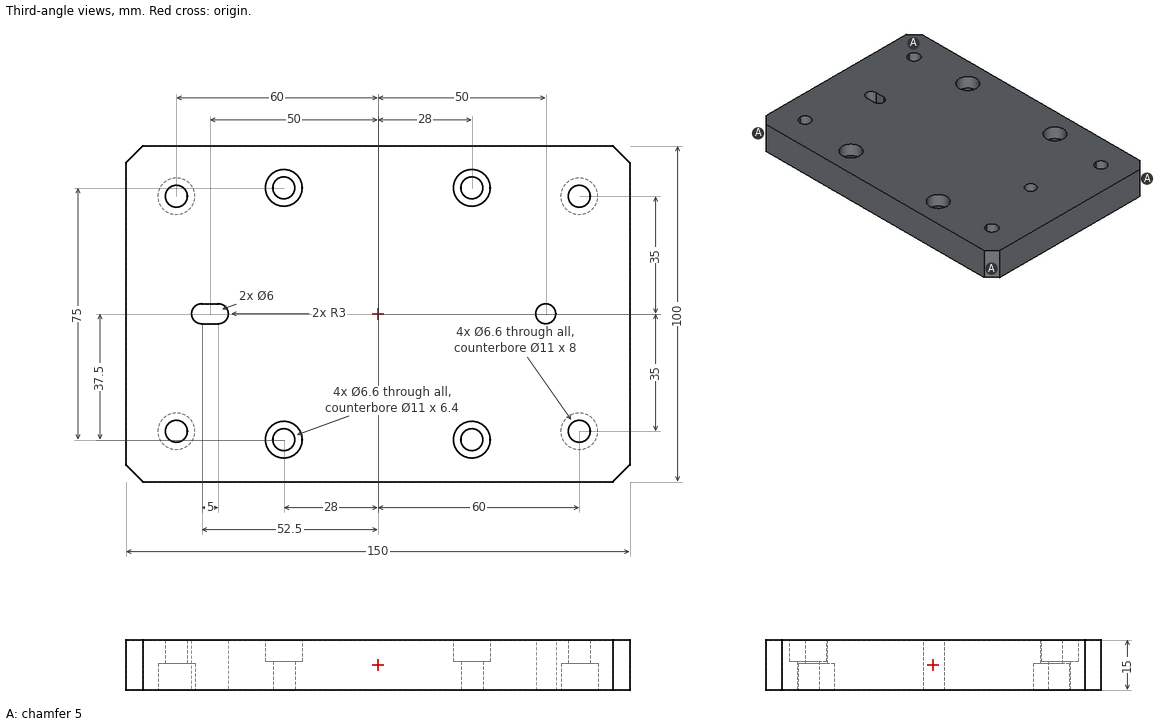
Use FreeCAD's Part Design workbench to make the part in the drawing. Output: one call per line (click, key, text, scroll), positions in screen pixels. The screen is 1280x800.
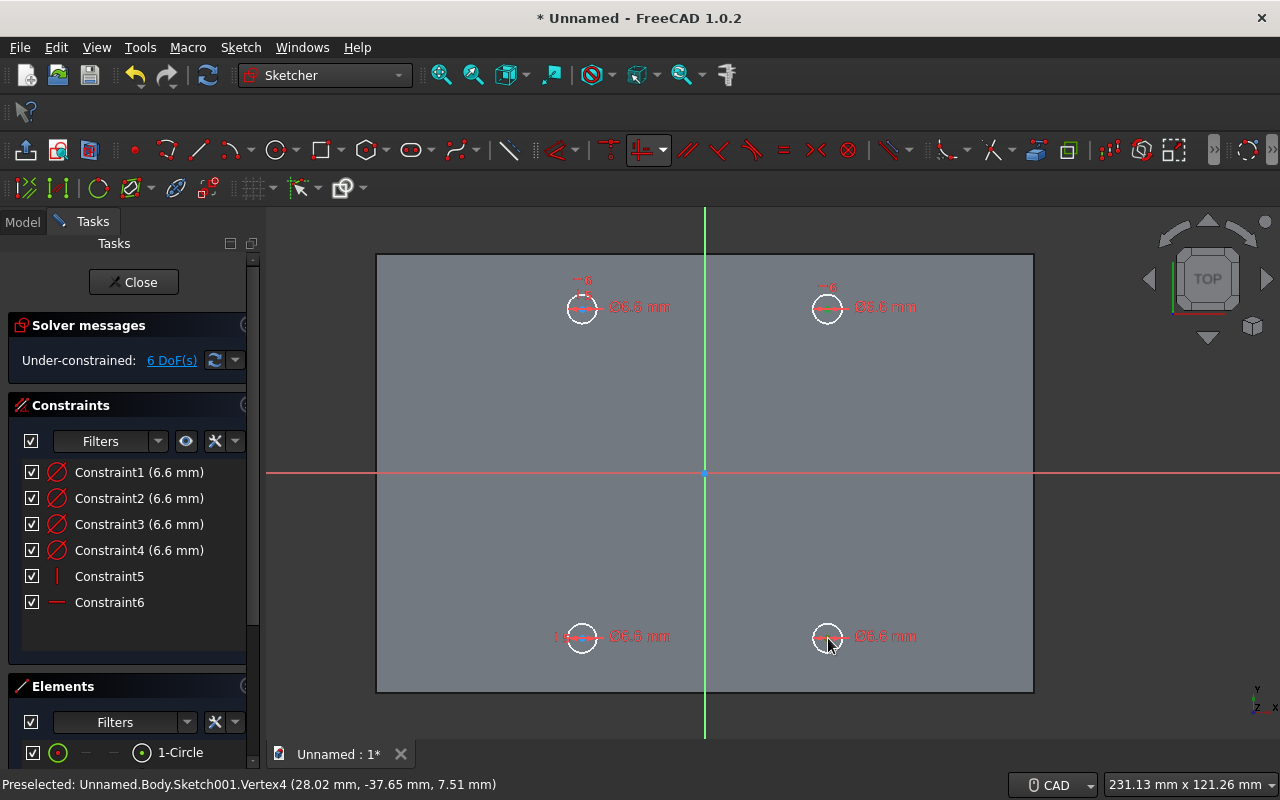
click(666, 150)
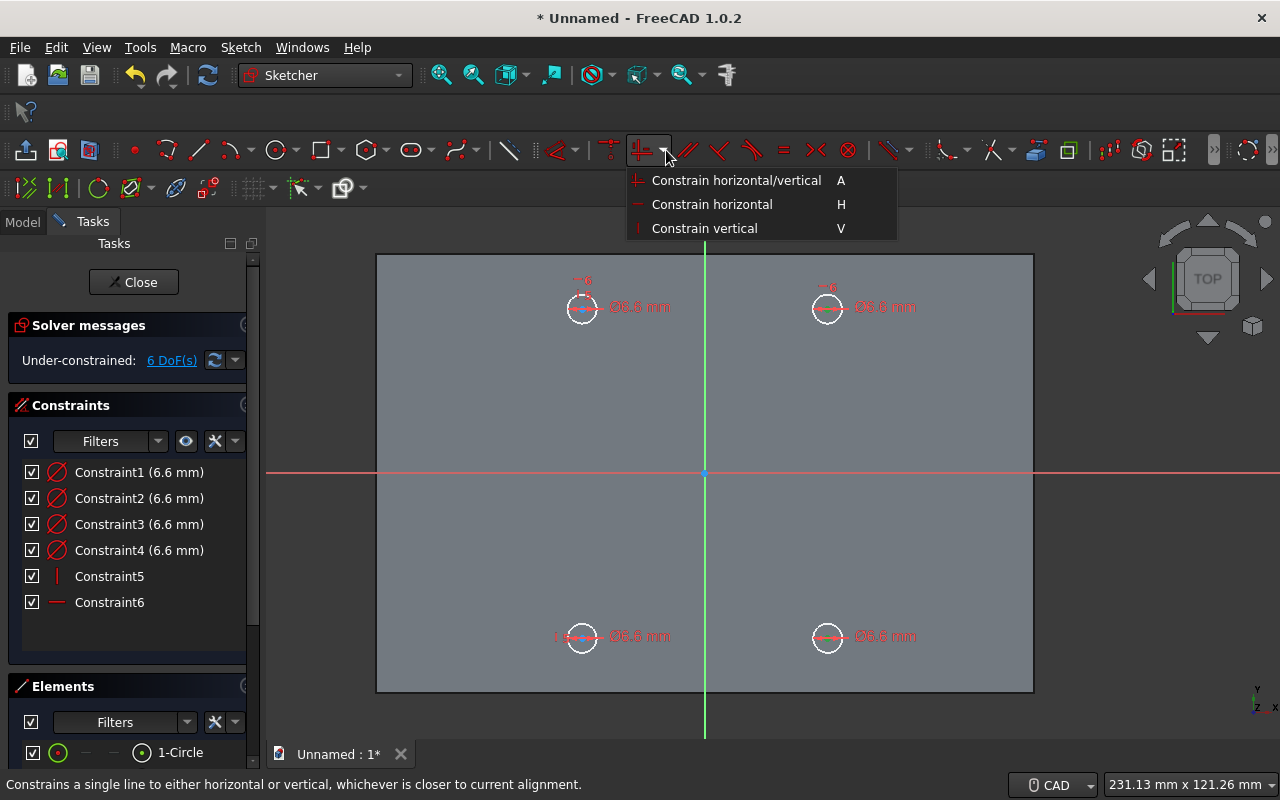
click(762, 228)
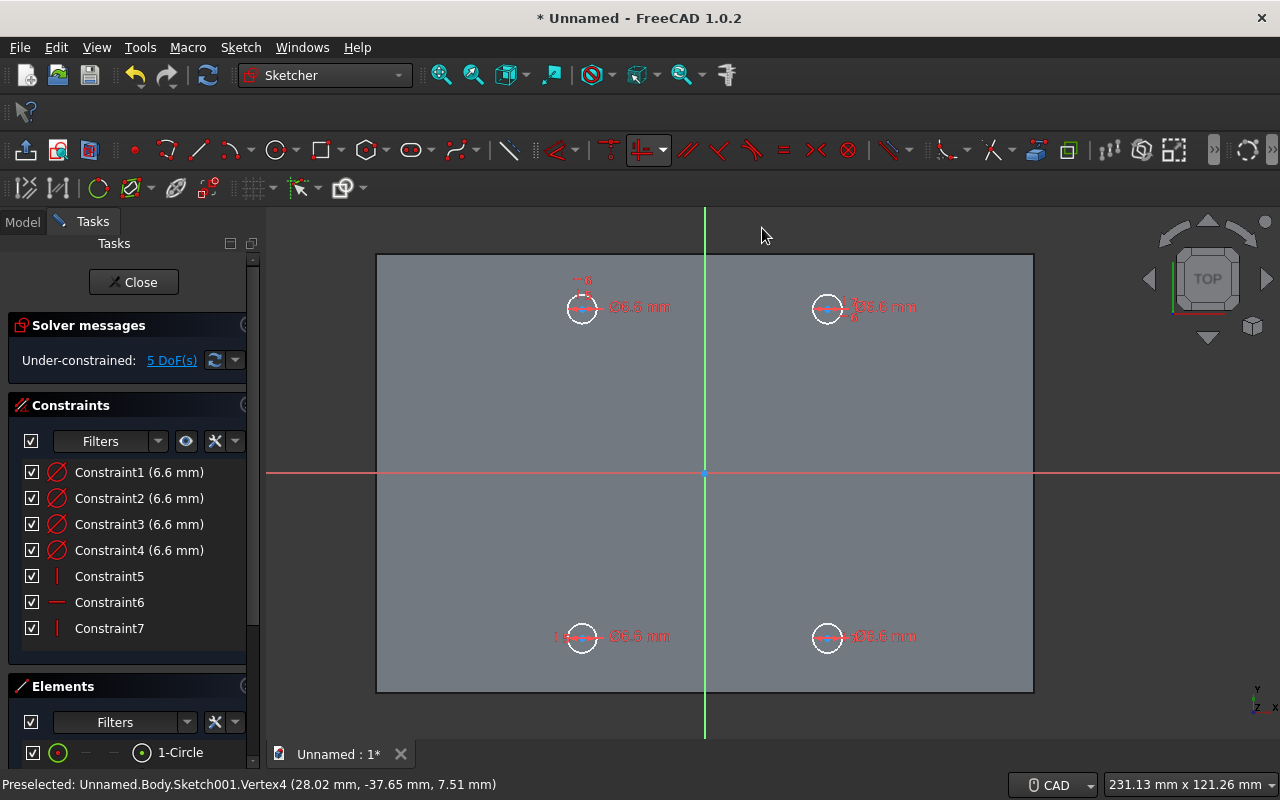
click(582, 638)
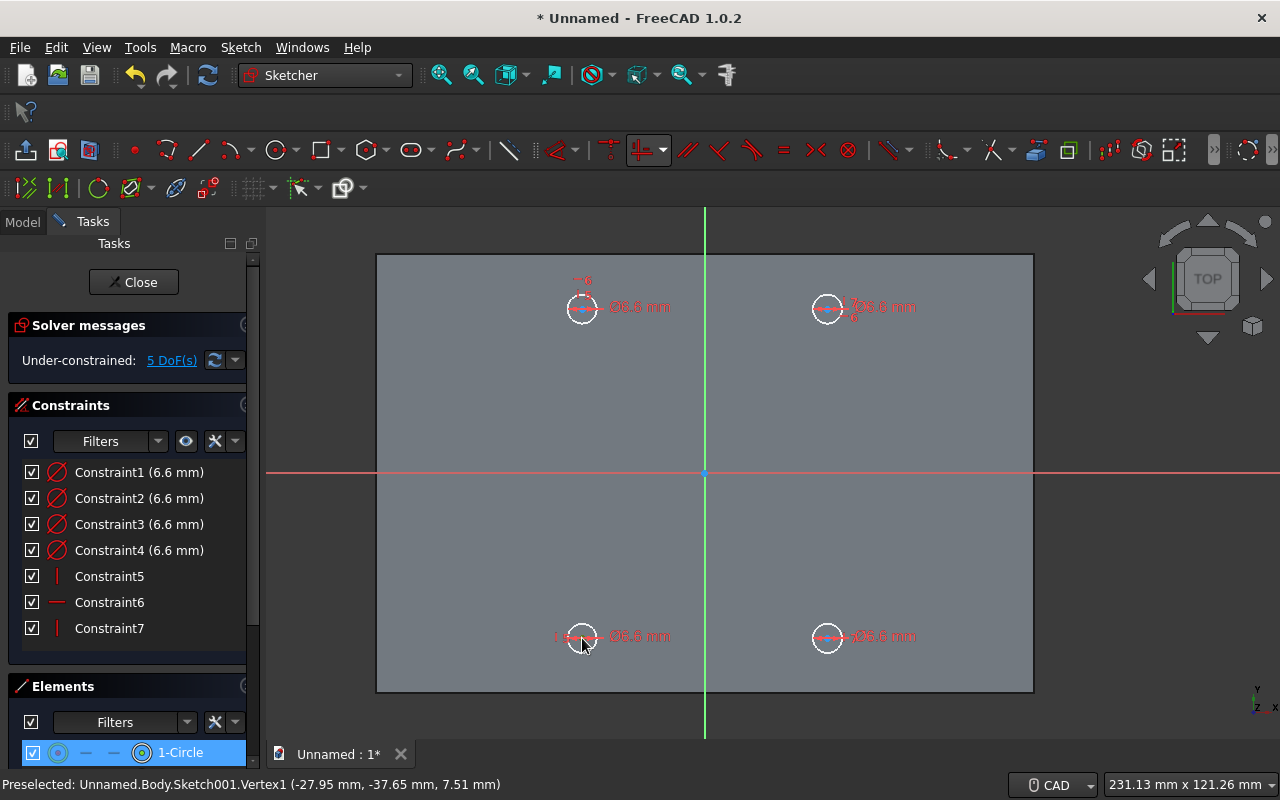
click(827, 638)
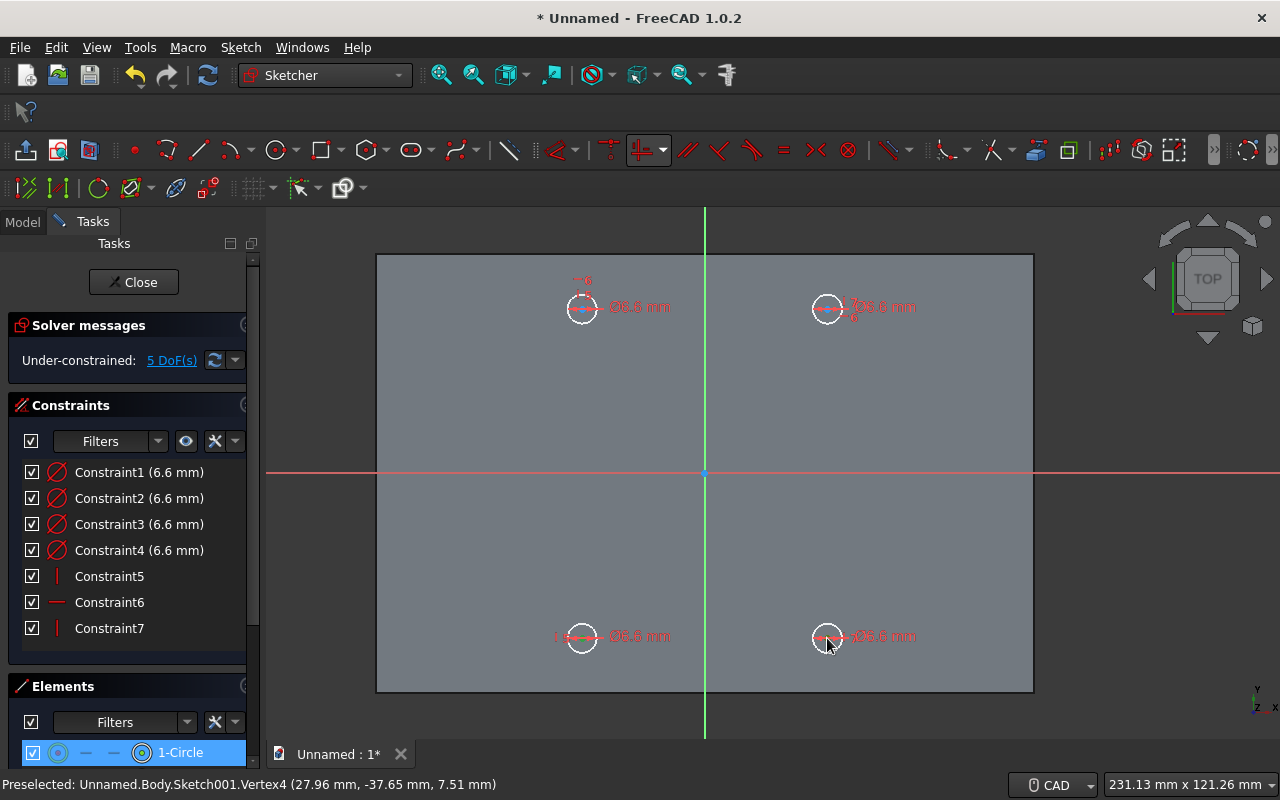
key(h)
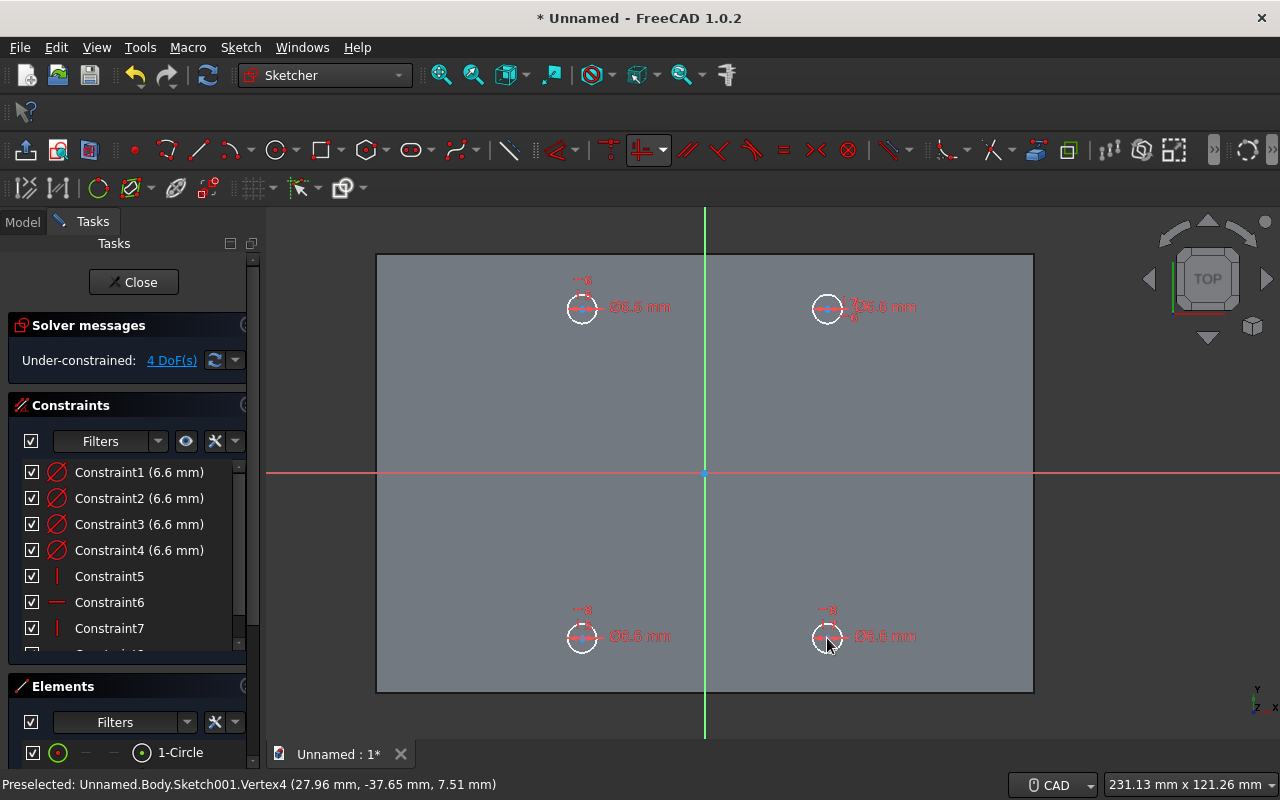
key(d)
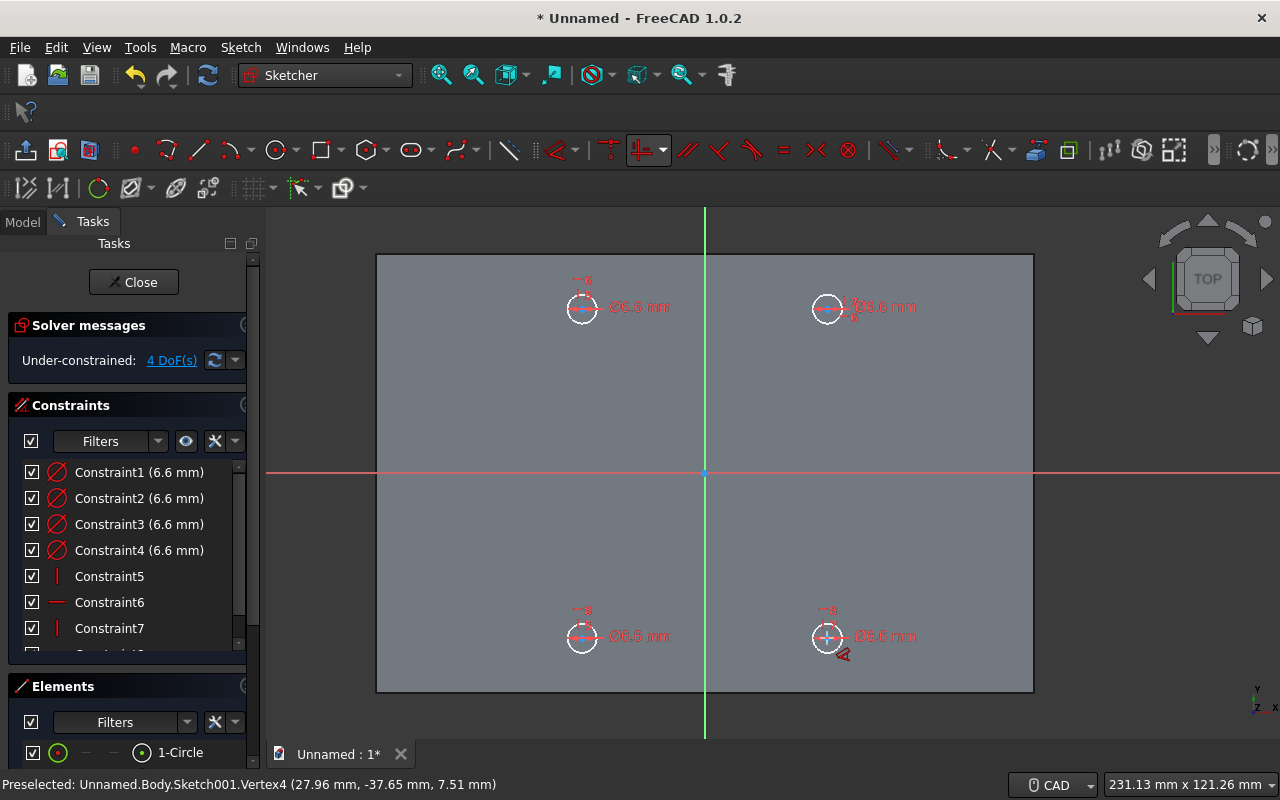
click(582, 638)
click(643, 672)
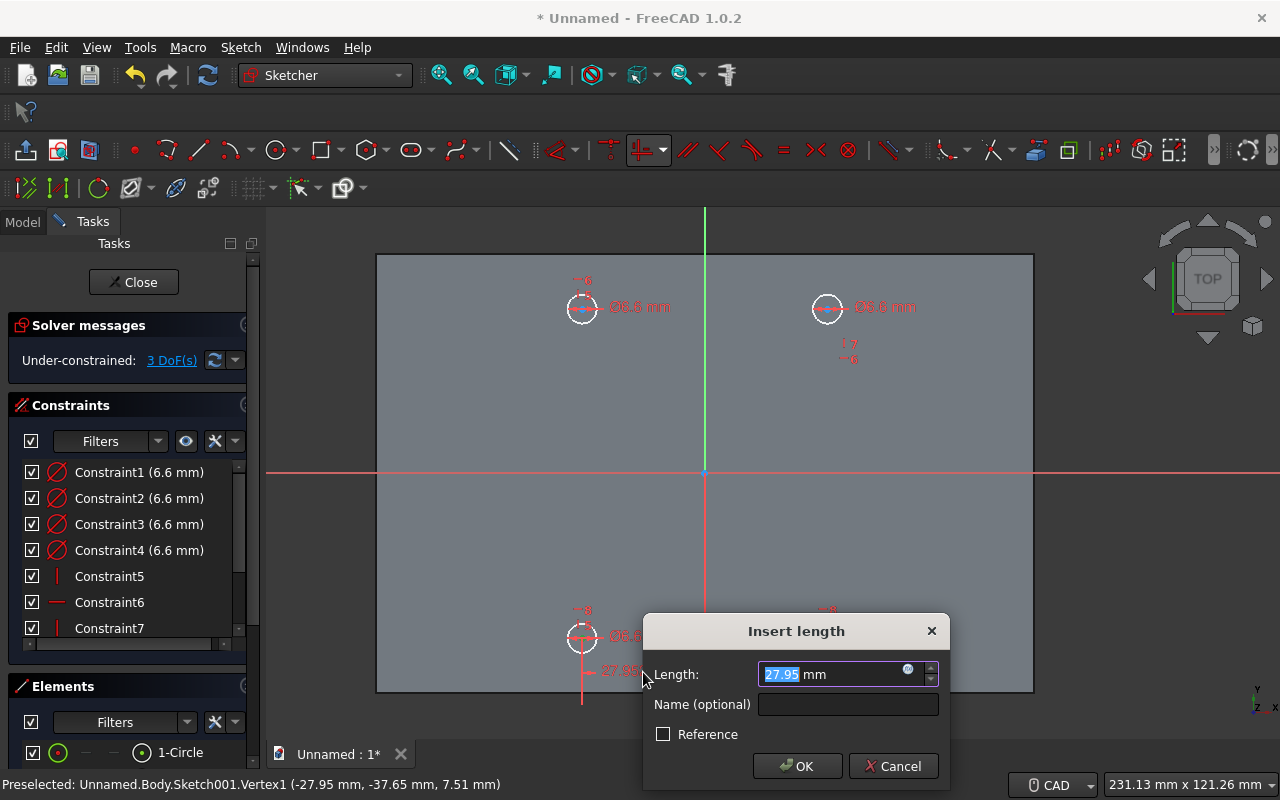
text(28)
key(Return)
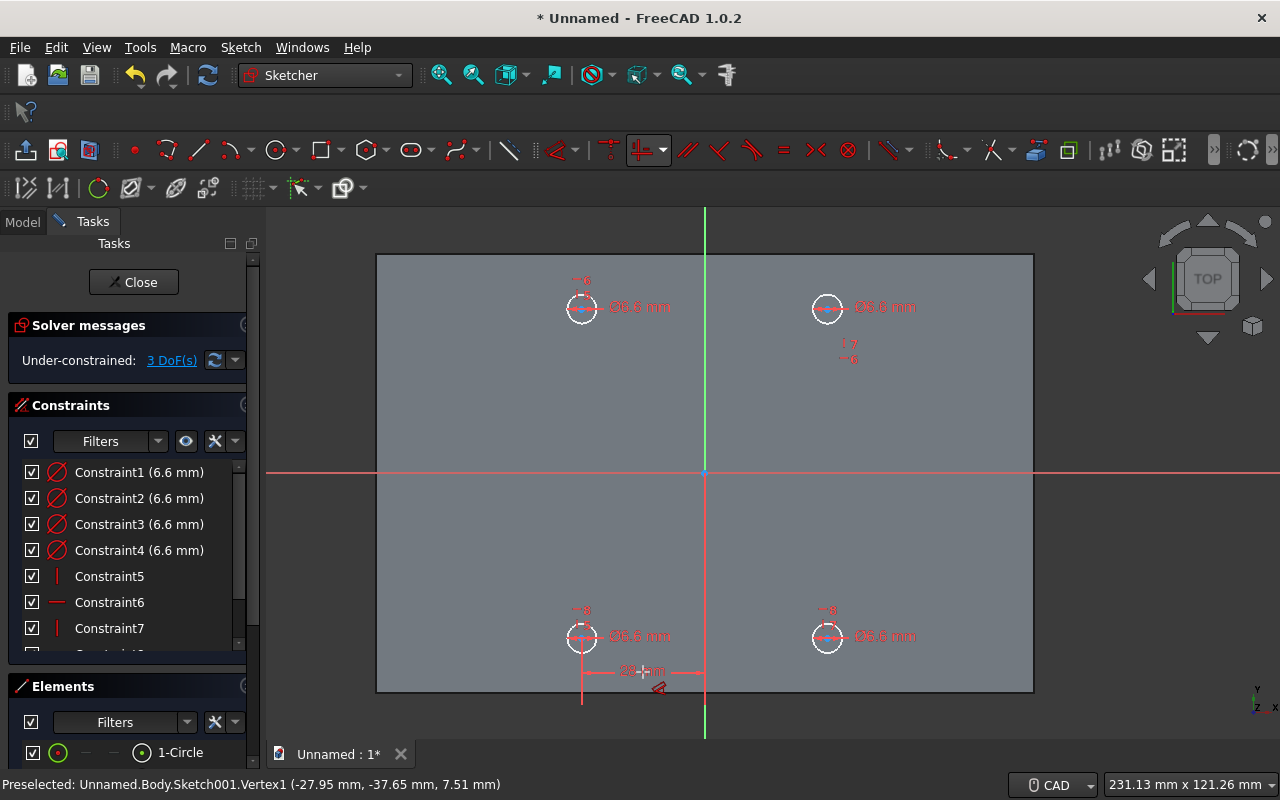
click(827, 309)
click(766, 275)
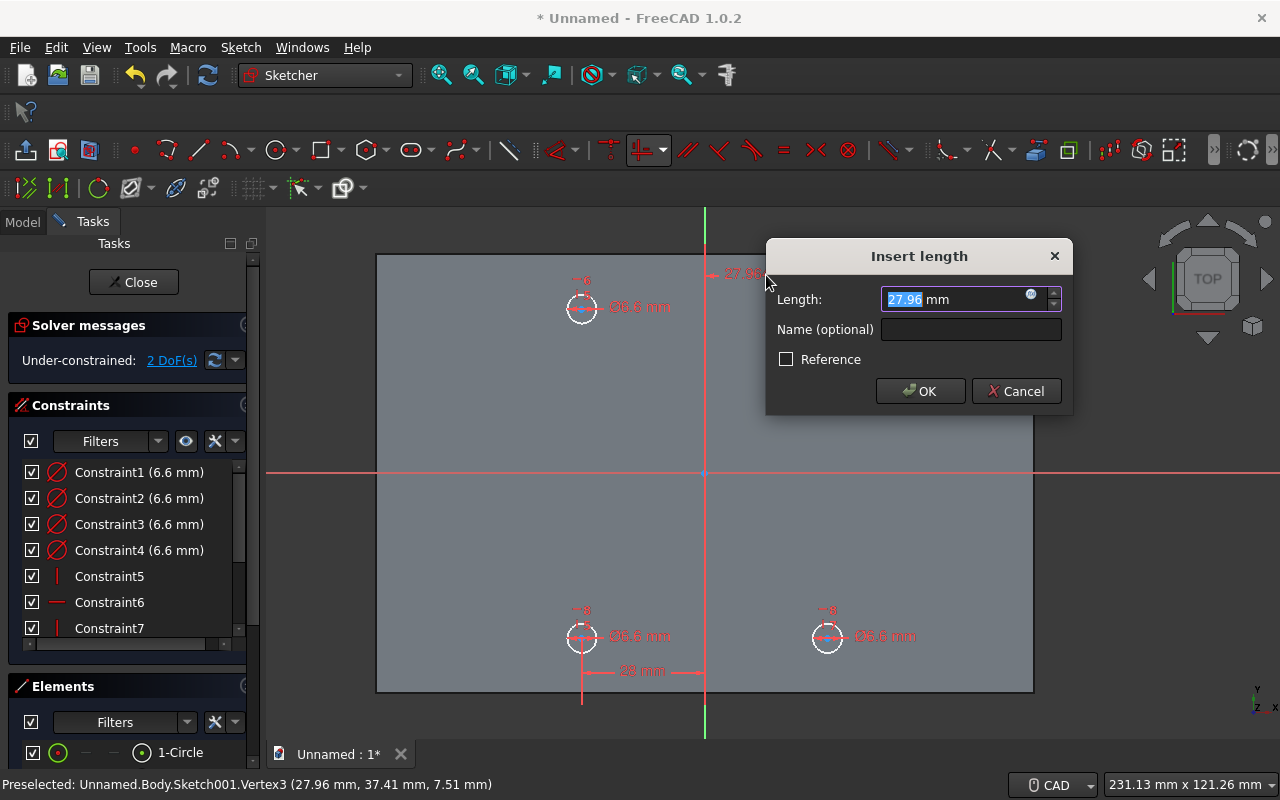
text(28)
key(Return)